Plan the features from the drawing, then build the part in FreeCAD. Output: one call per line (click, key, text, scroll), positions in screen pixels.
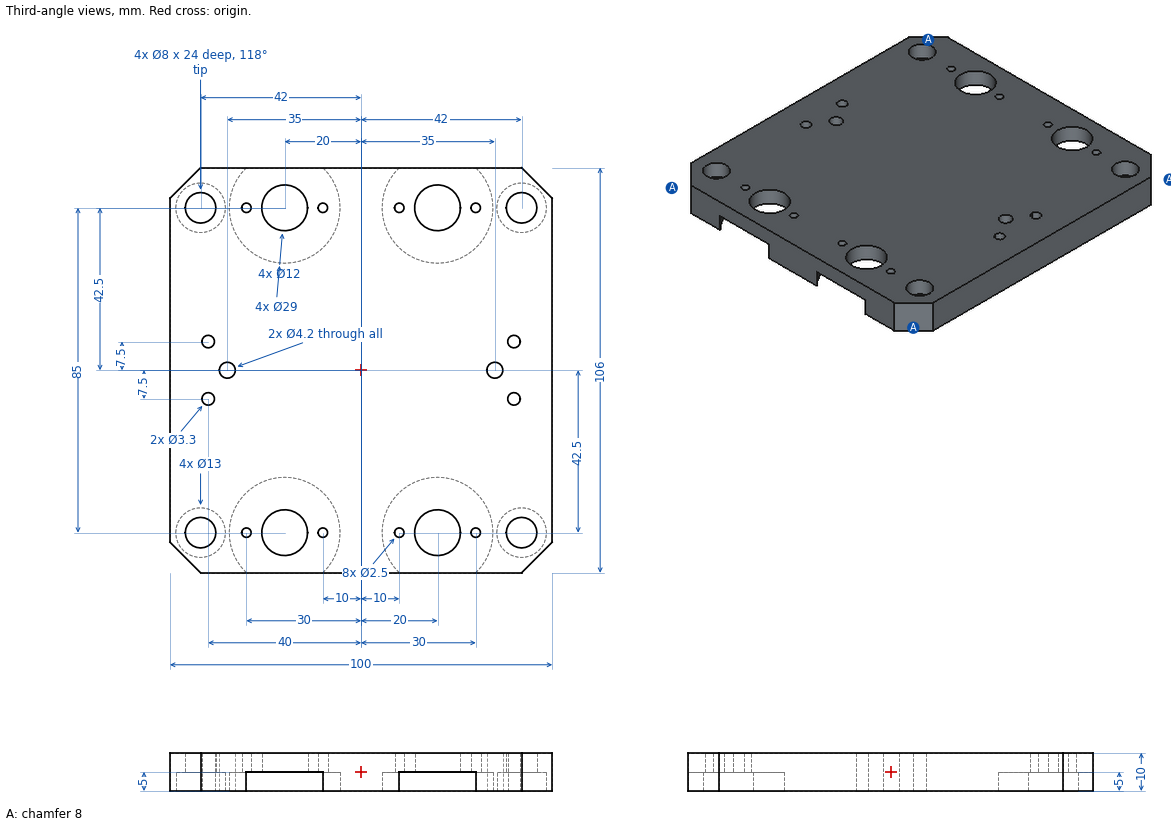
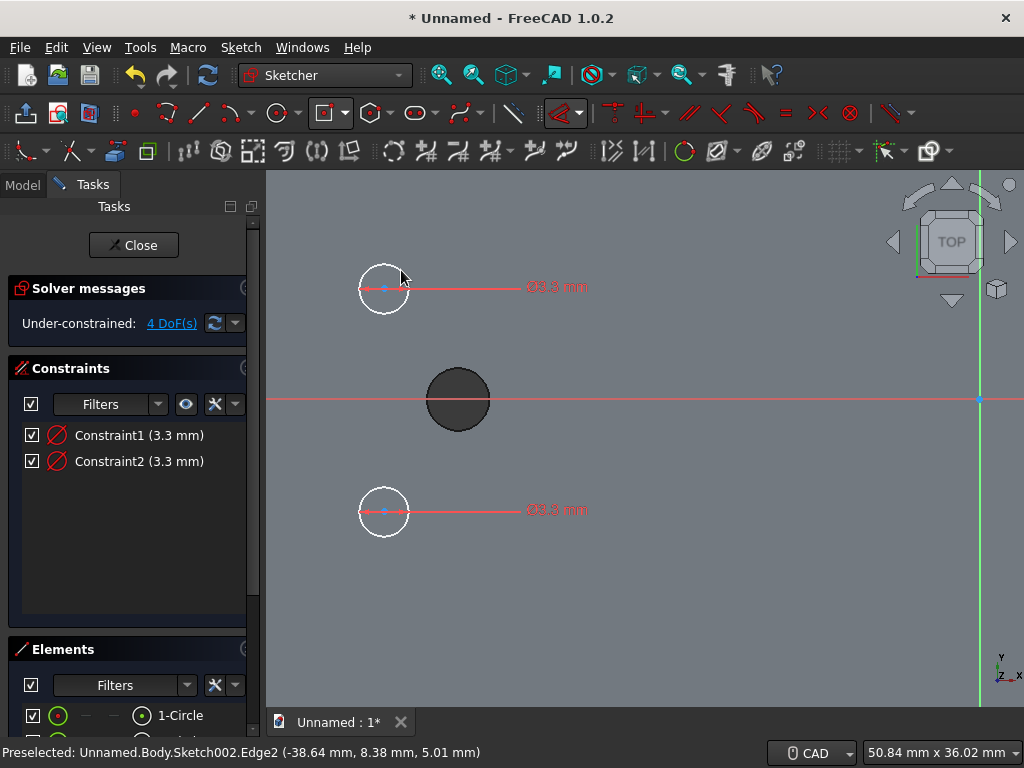
click(384, 512)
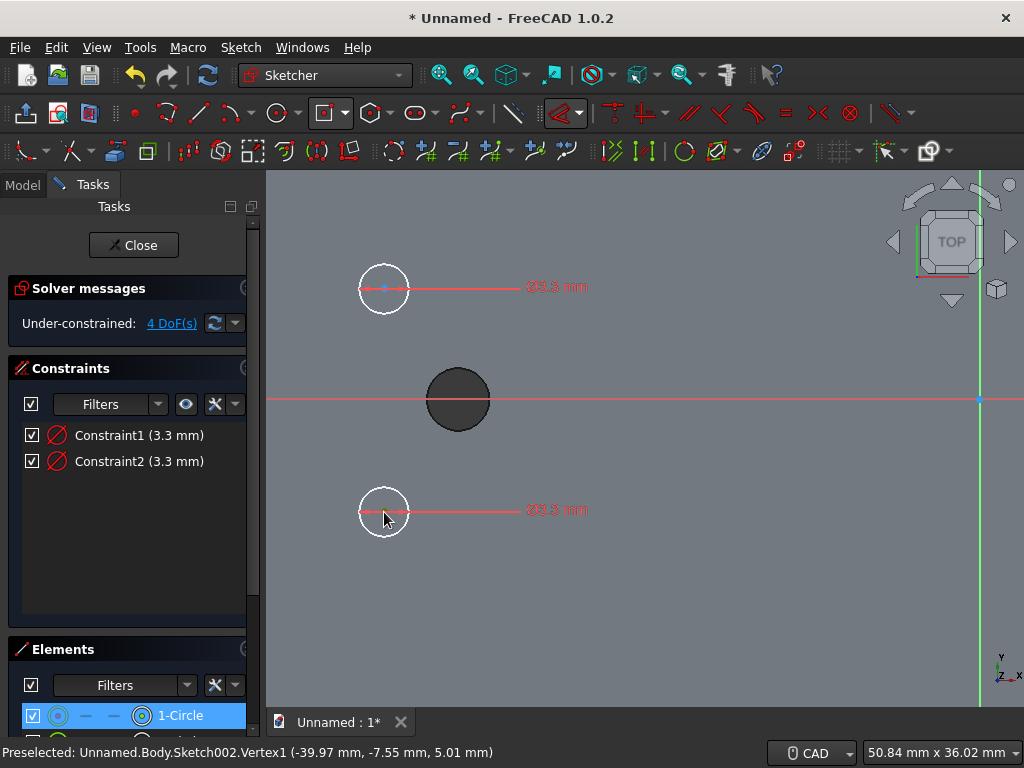
click(384, 289)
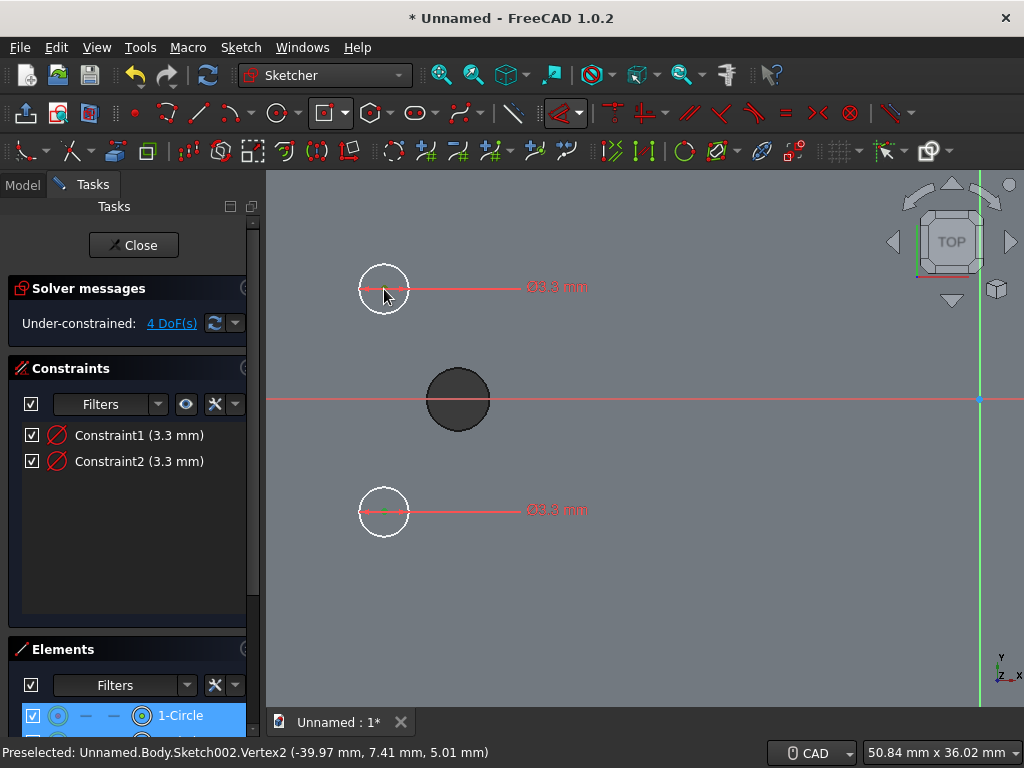
click(668, 114)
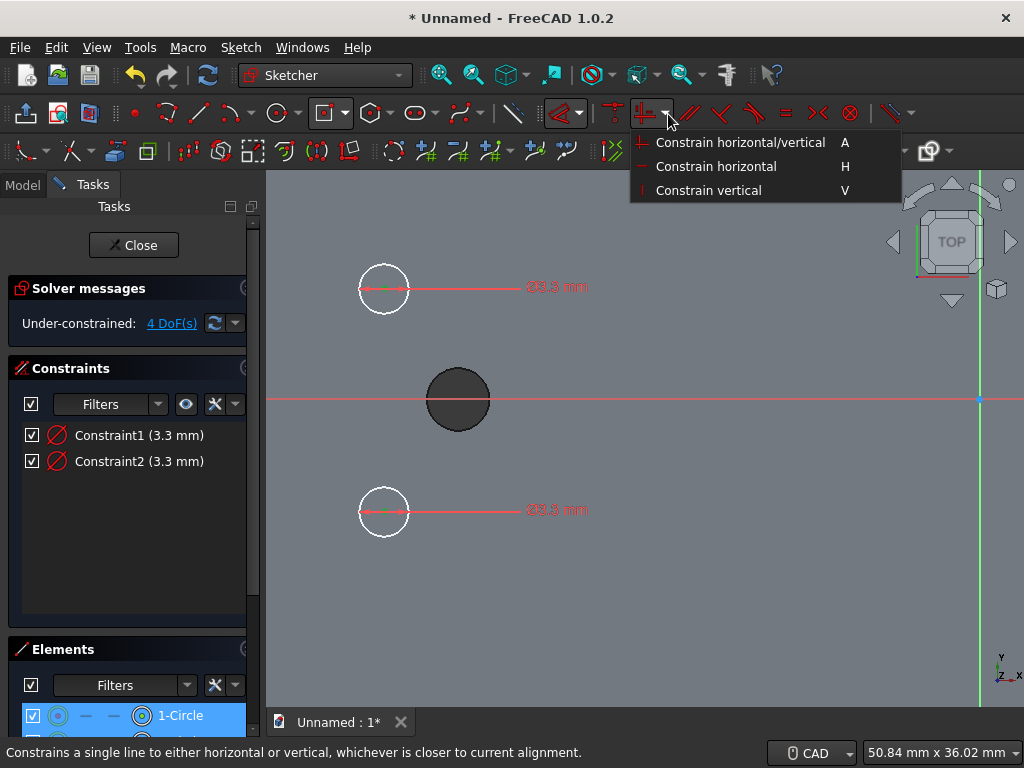
click(766, 190)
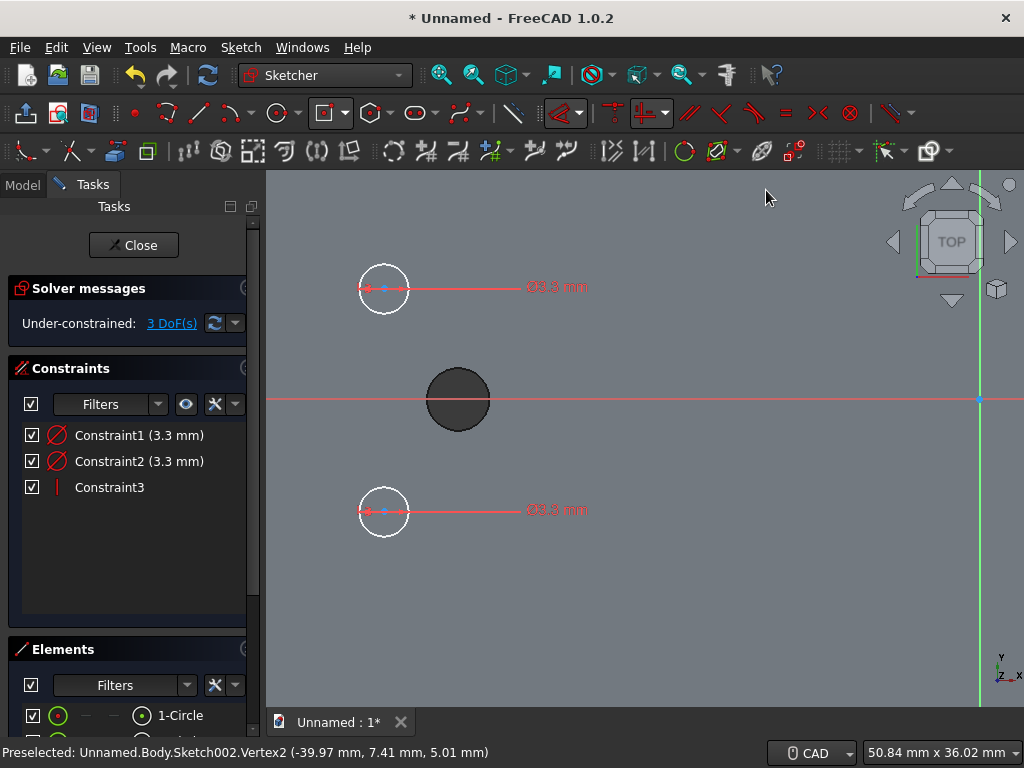
click(384, 512)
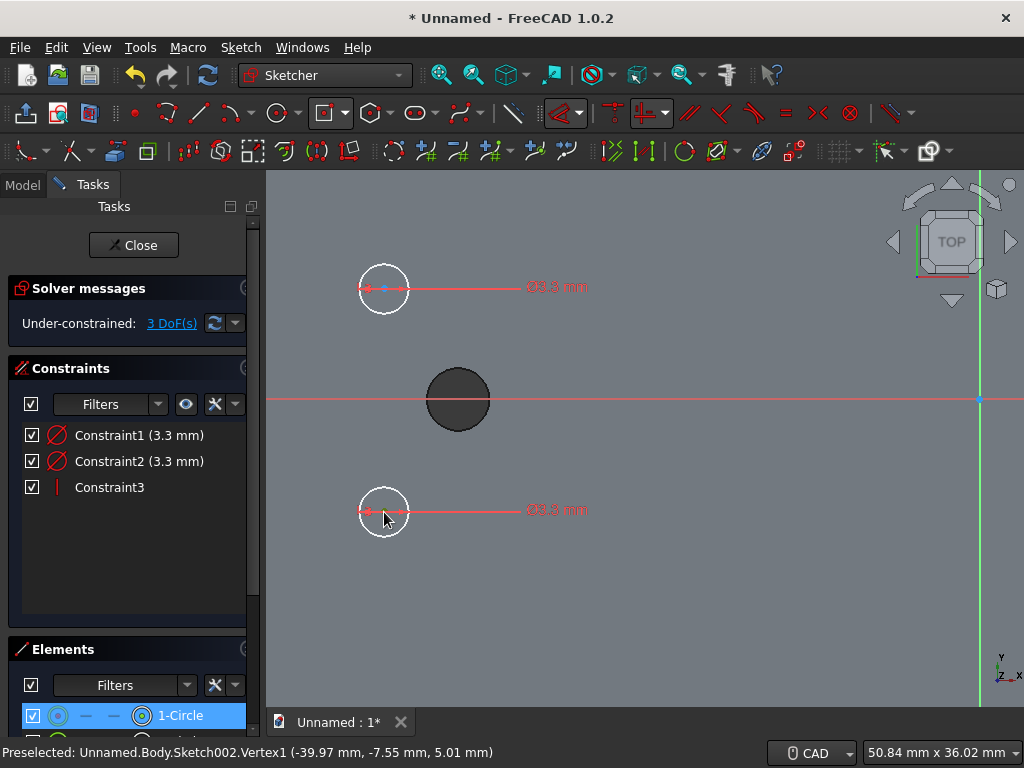
click(582, 114)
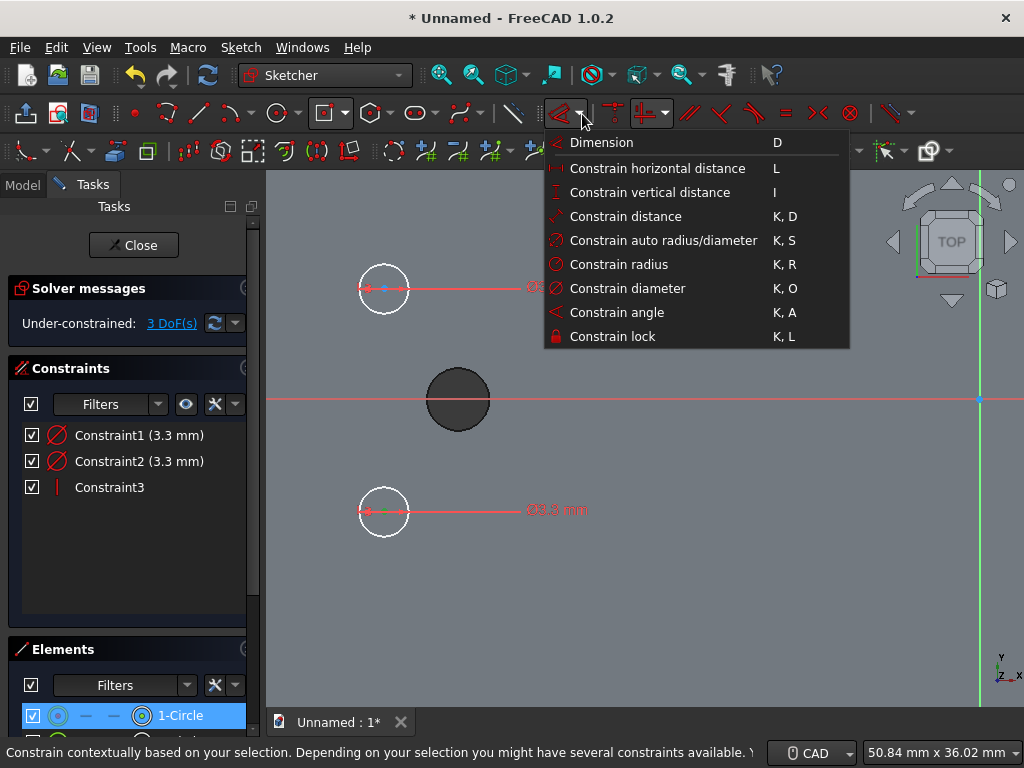
click(697, 168)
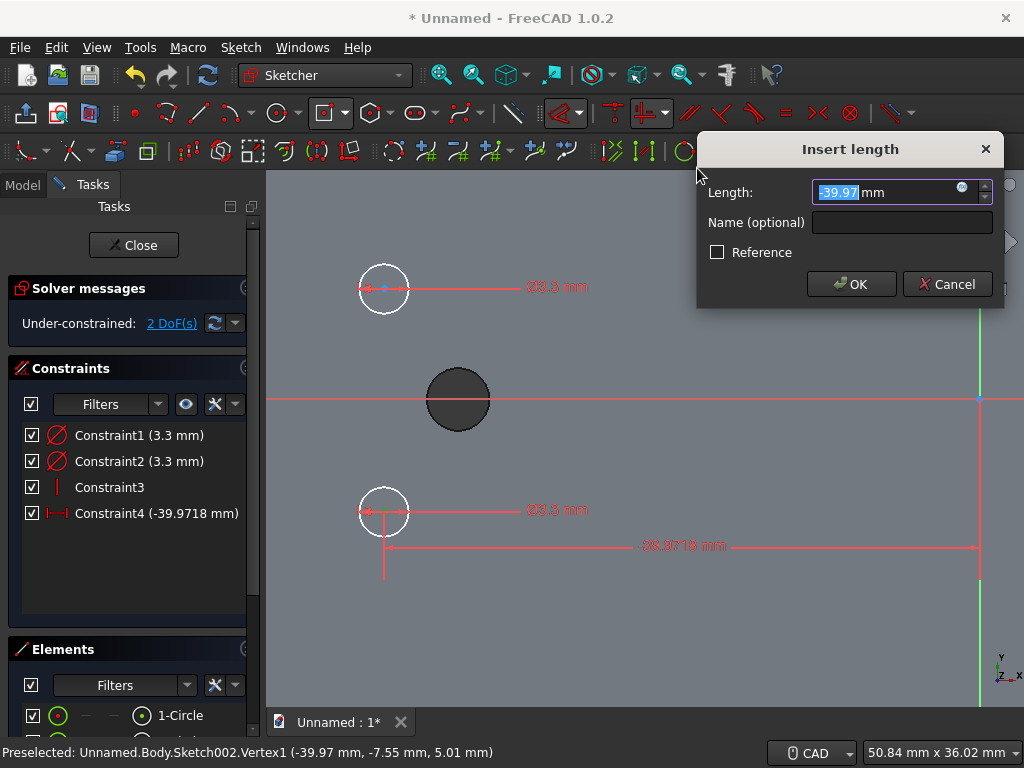
text(-40)
key(Return)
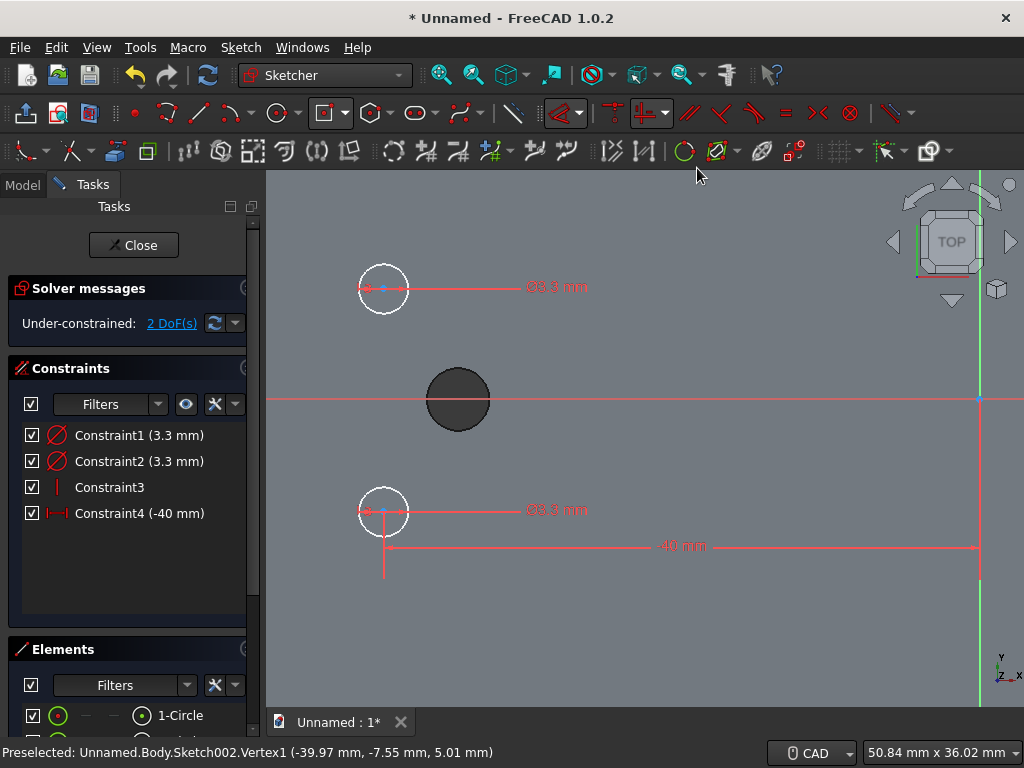
click(384, 512)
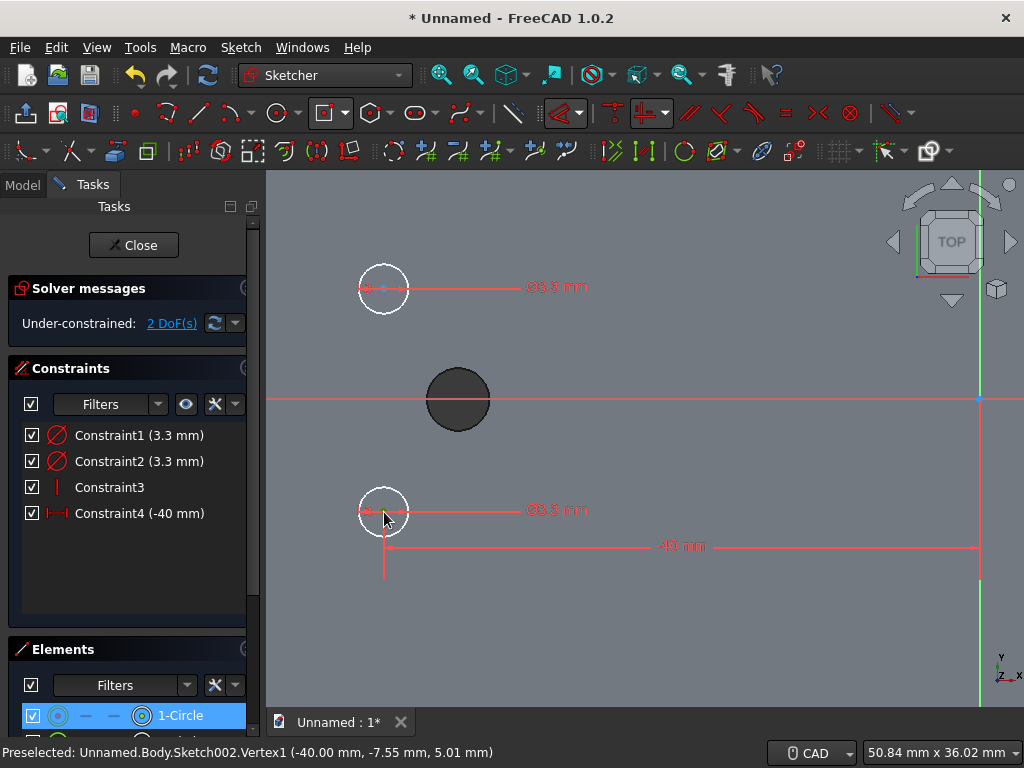
key(i)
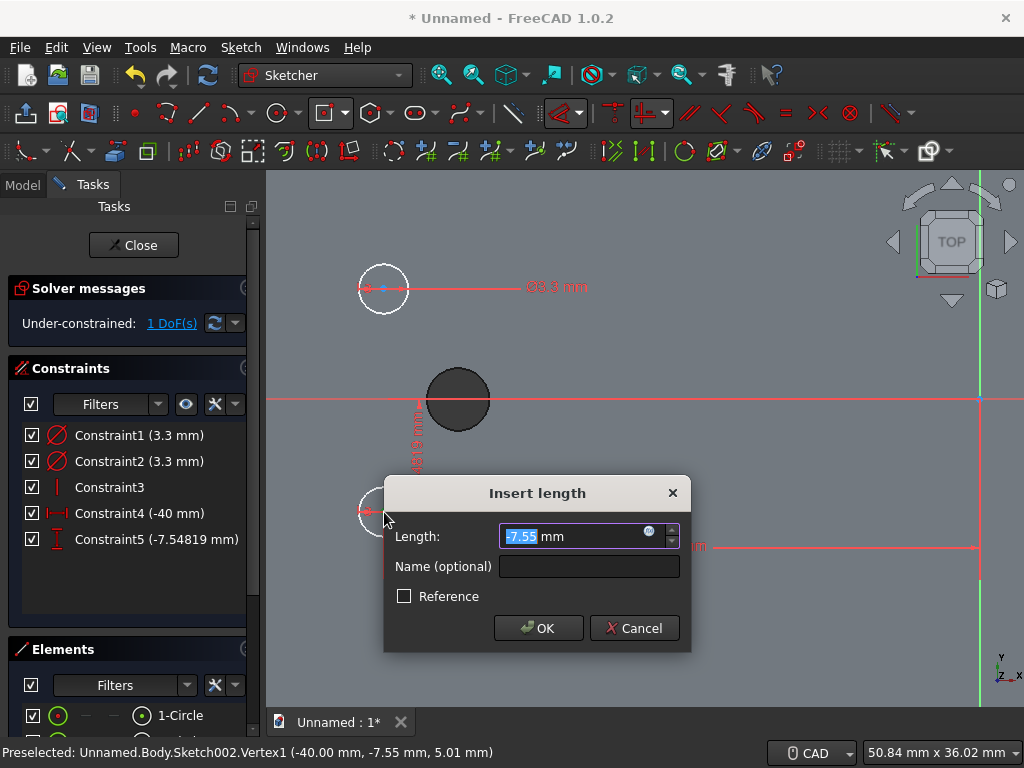
text(-7.5)
key(Return)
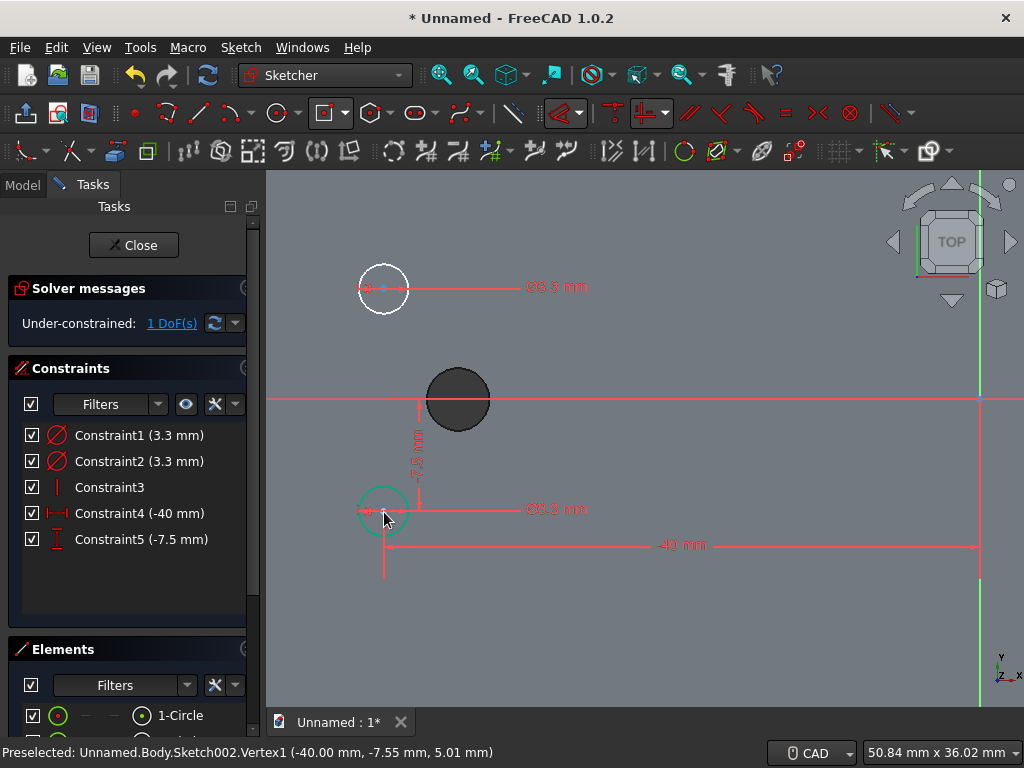
click(384, 289)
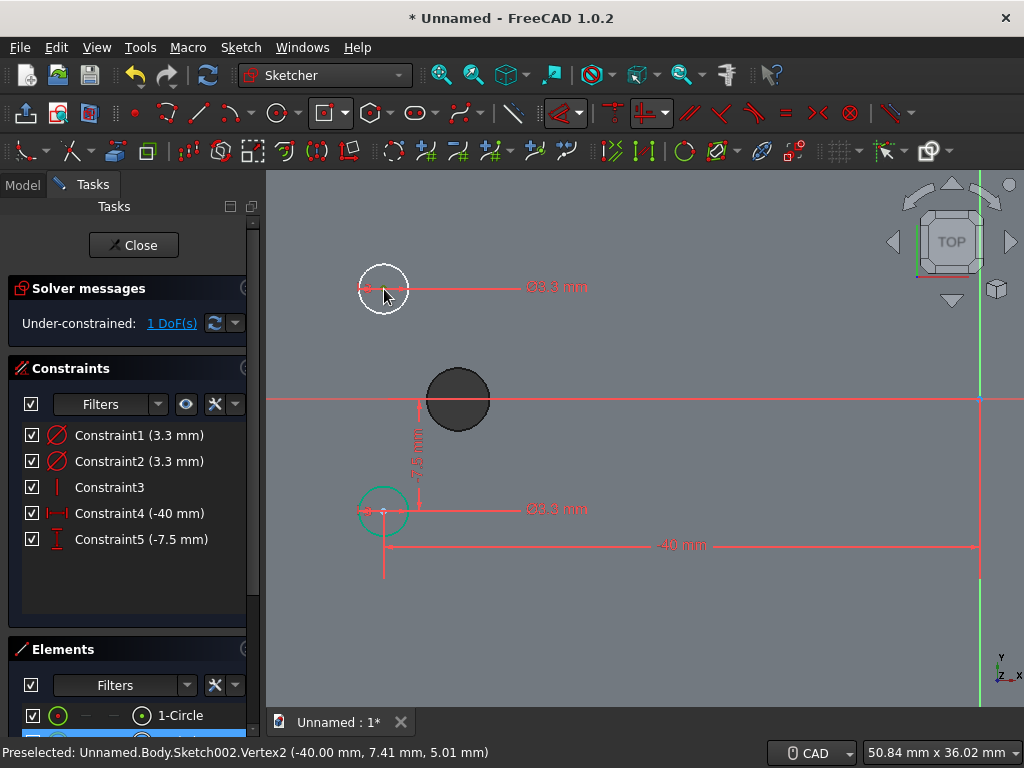
key(i)